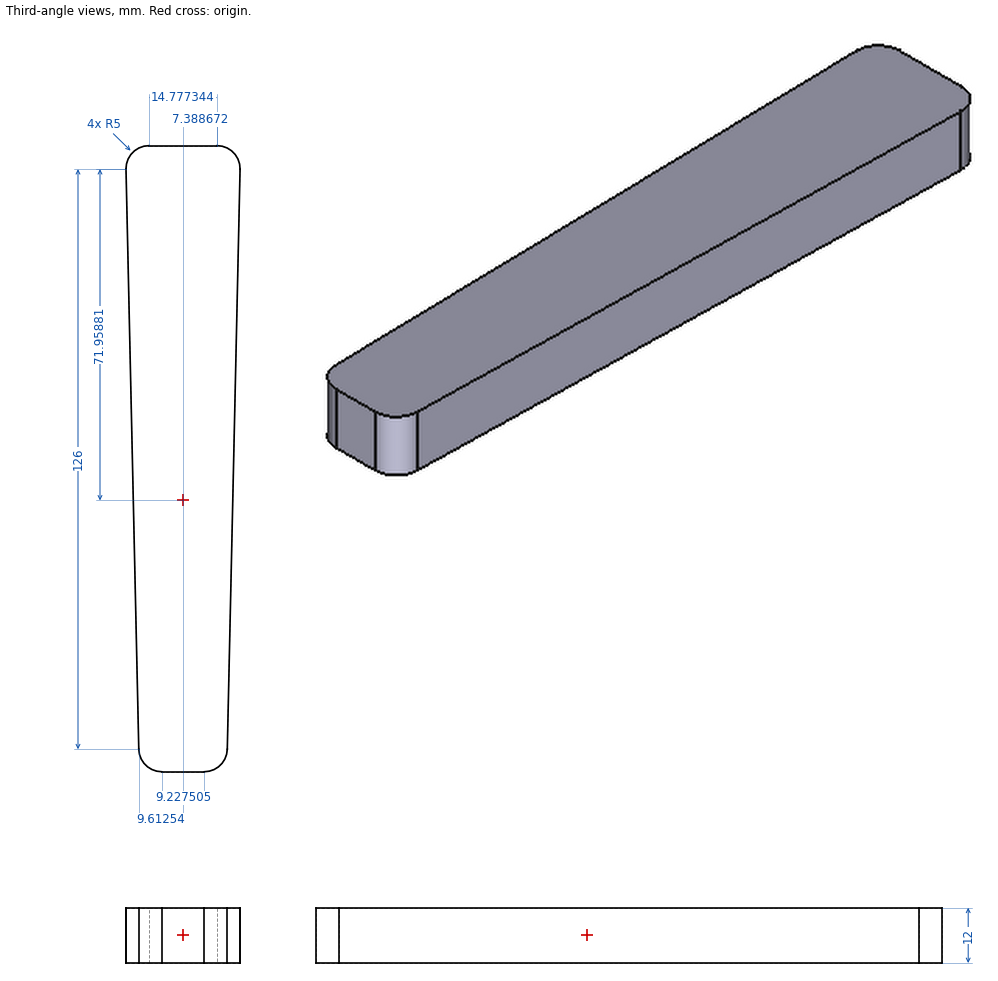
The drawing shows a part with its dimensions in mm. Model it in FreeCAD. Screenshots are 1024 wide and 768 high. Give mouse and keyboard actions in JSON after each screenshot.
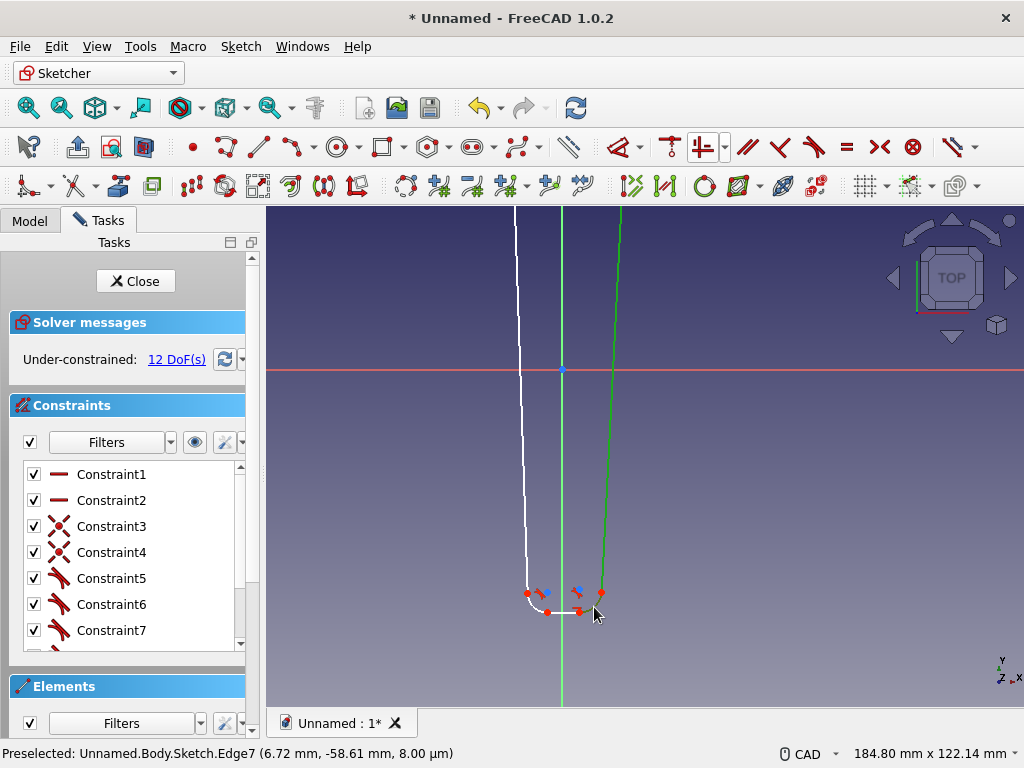
{"action": "key", "text": "t"}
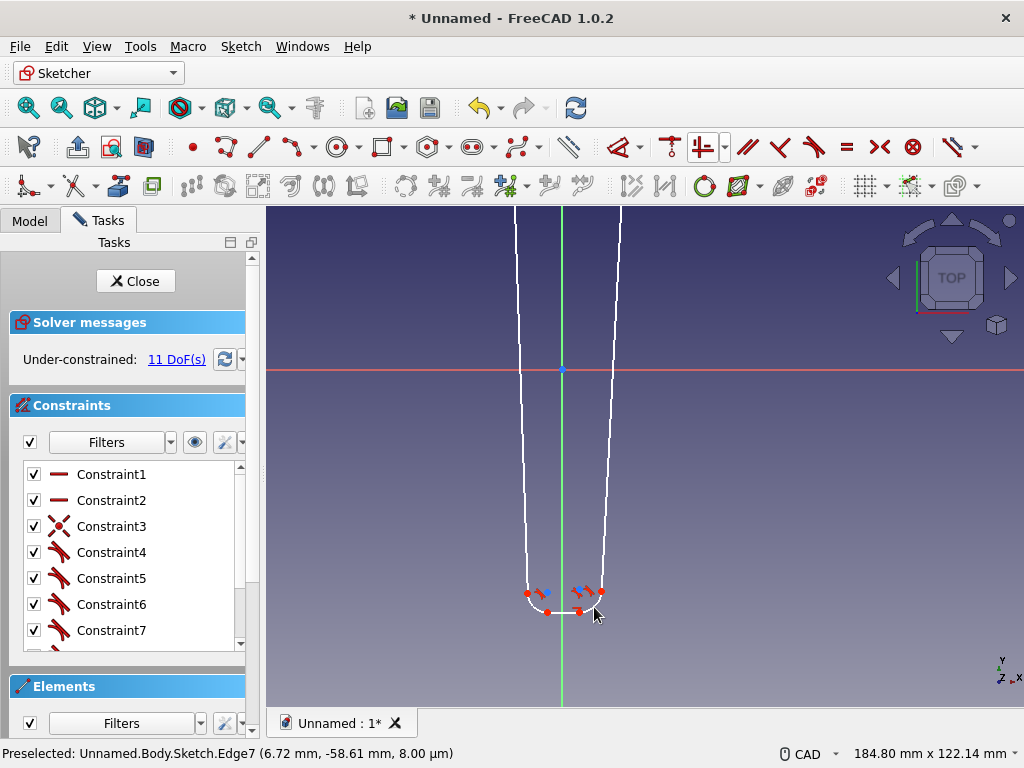
{"action": "left_click", "coordinate": [610, 436]}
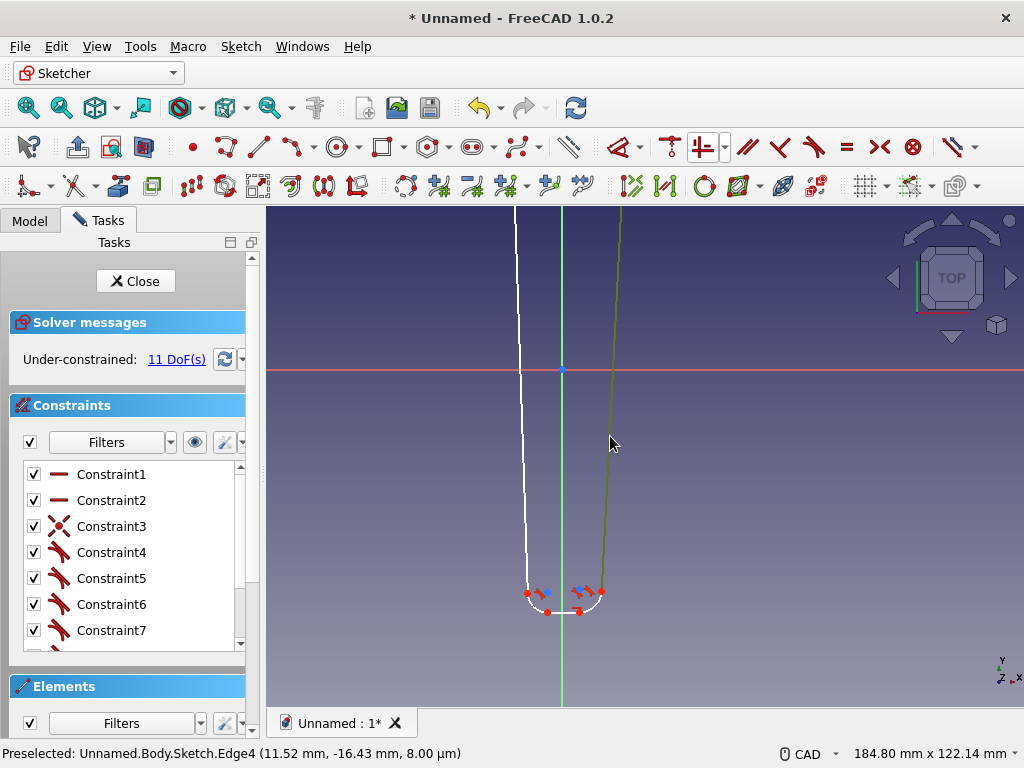
{"action": "scroll", "coordinate": [594, 607], "scroll_direction": "down", "scroll_amount": 3}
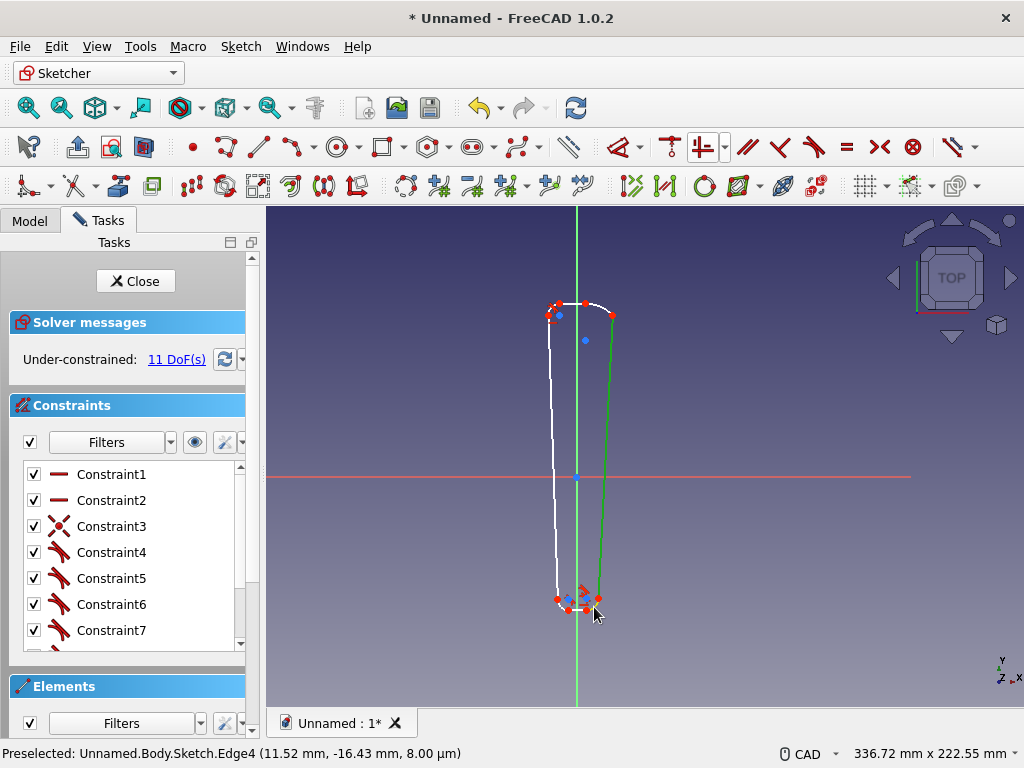
{"action": "scroll", "coordinate": [606, 310], "scroll_direction": "up", "scroll_amount": 3}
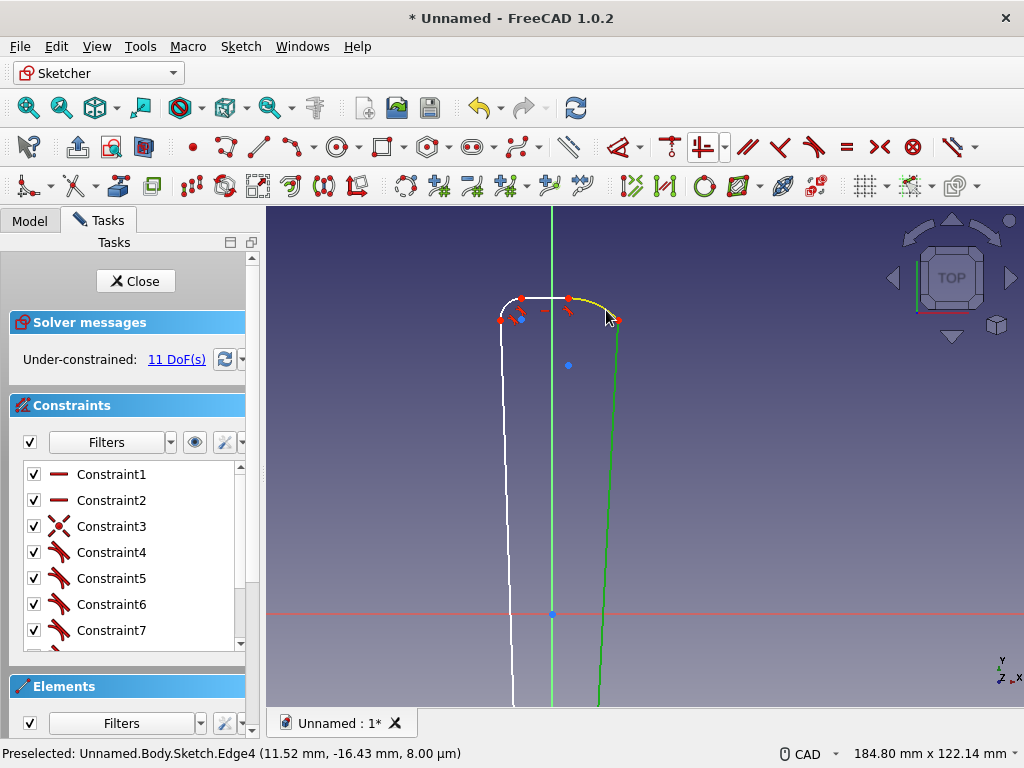
{"action": "left_click", "coordinate": [606, 309]}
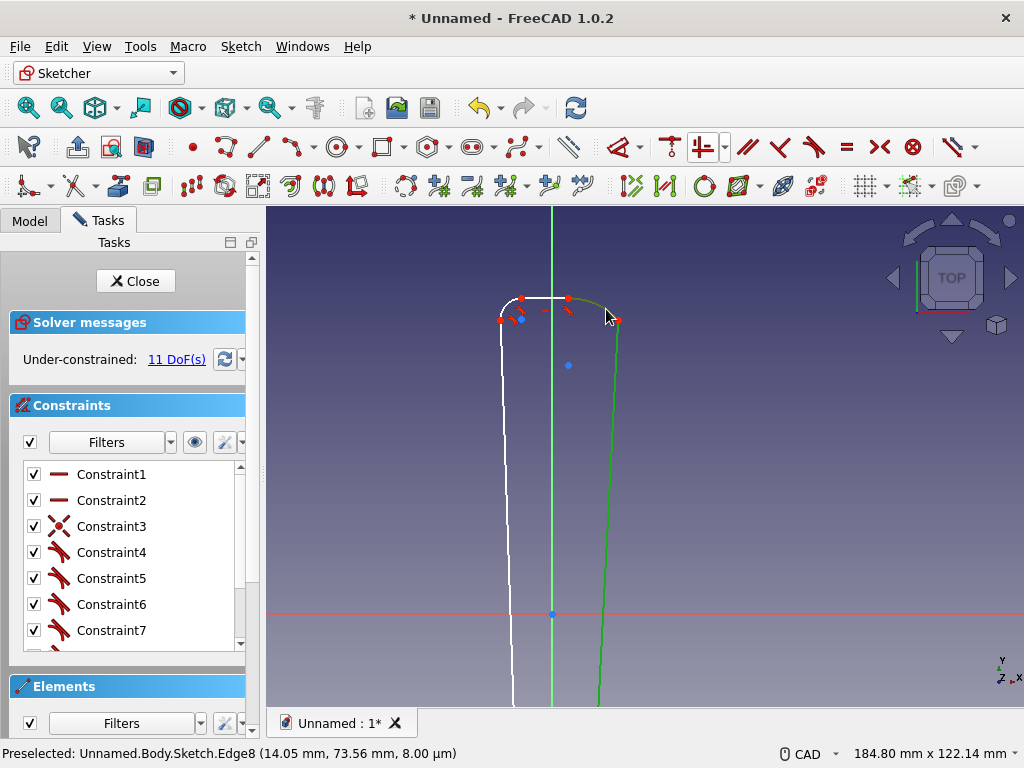
{"action": "key", "text": "t"}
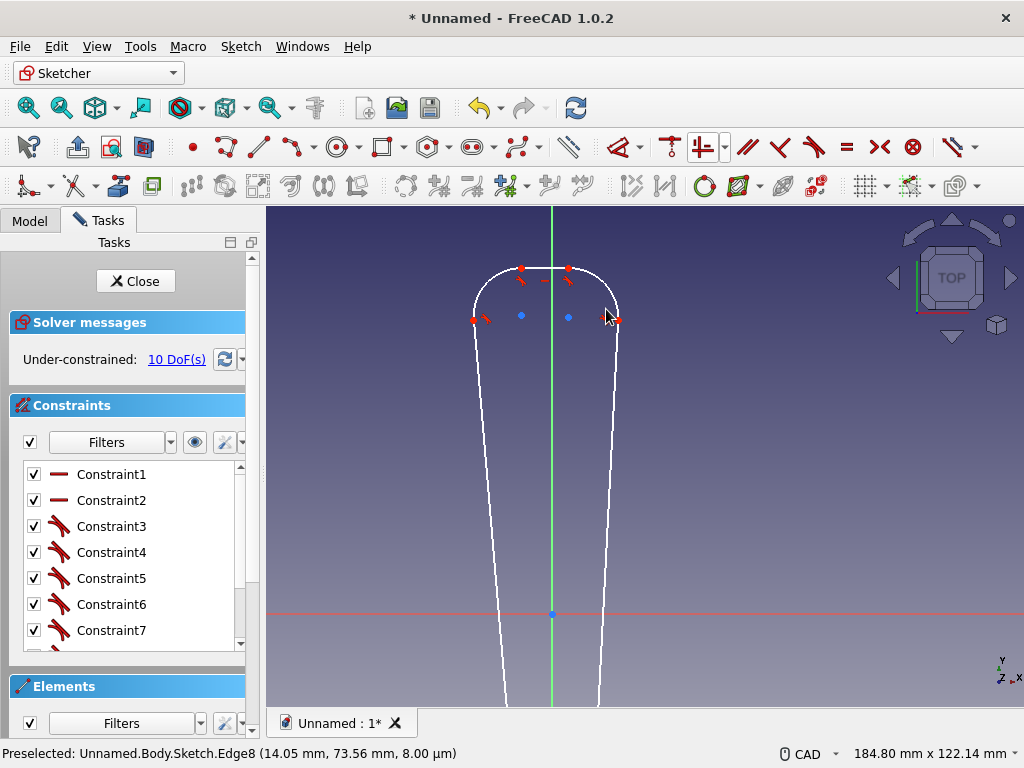
{"action": "left_click", "coordinate": [499, 274]}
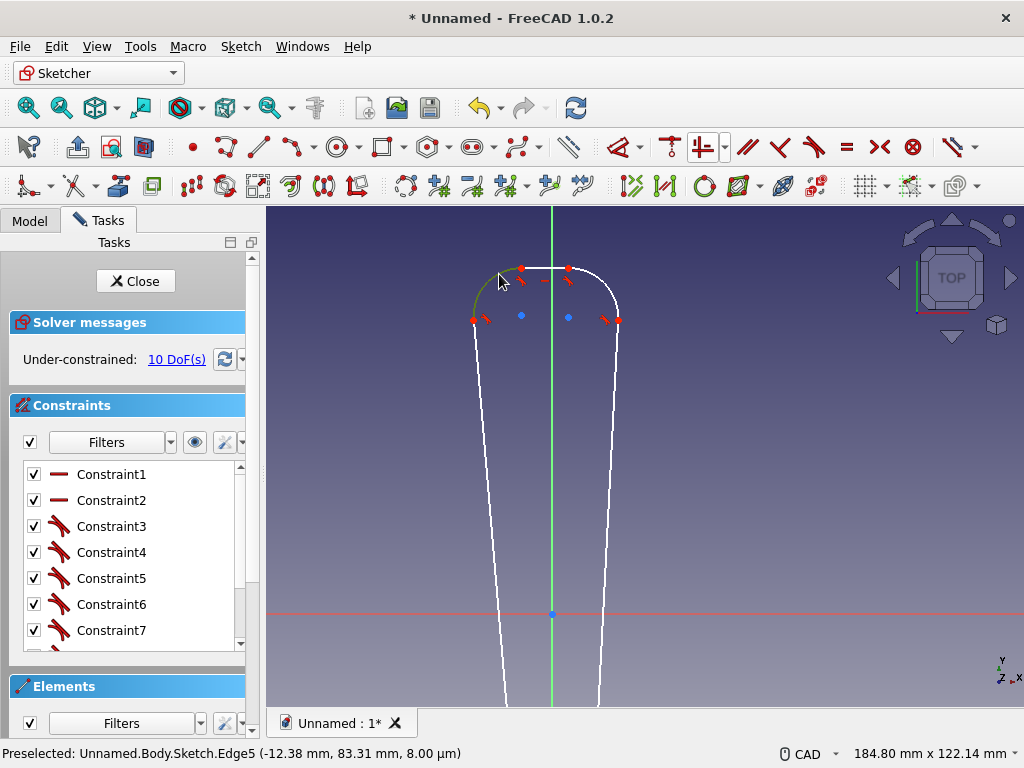
{"action": "scroll", "coordinate": [606, 310], "scroll_direction": "down", "scroll_amount": 3}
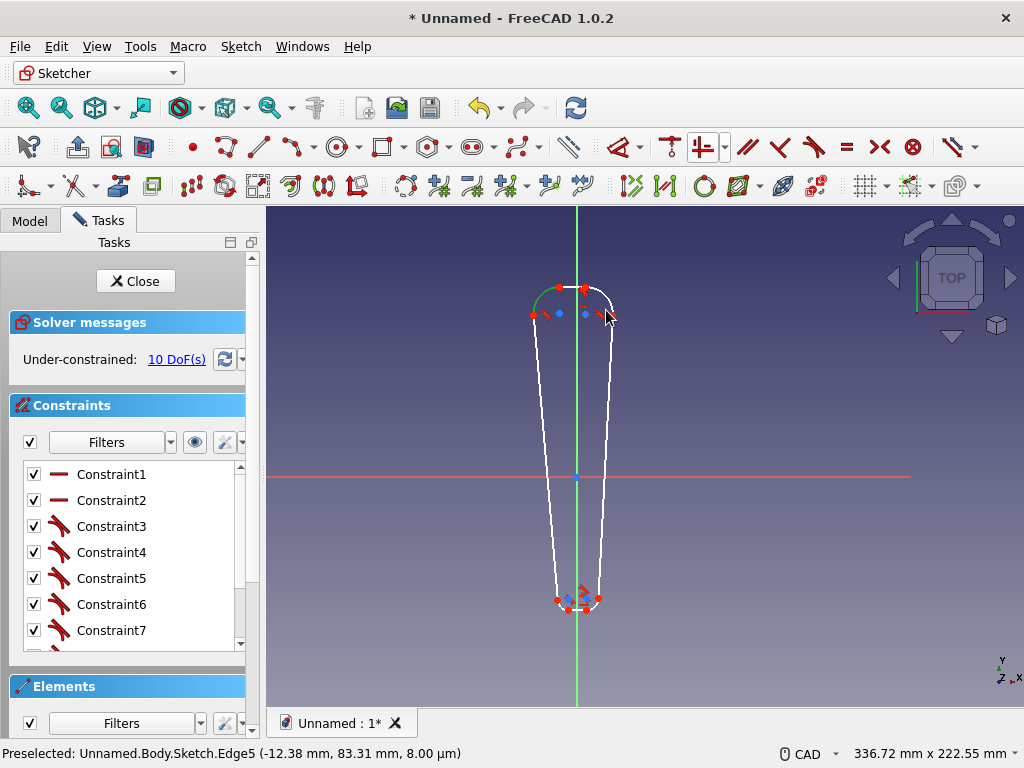
{"action": "scroll", "coordinate": [561, 608], "scroll_direction": "up", "scroll_amount": 3}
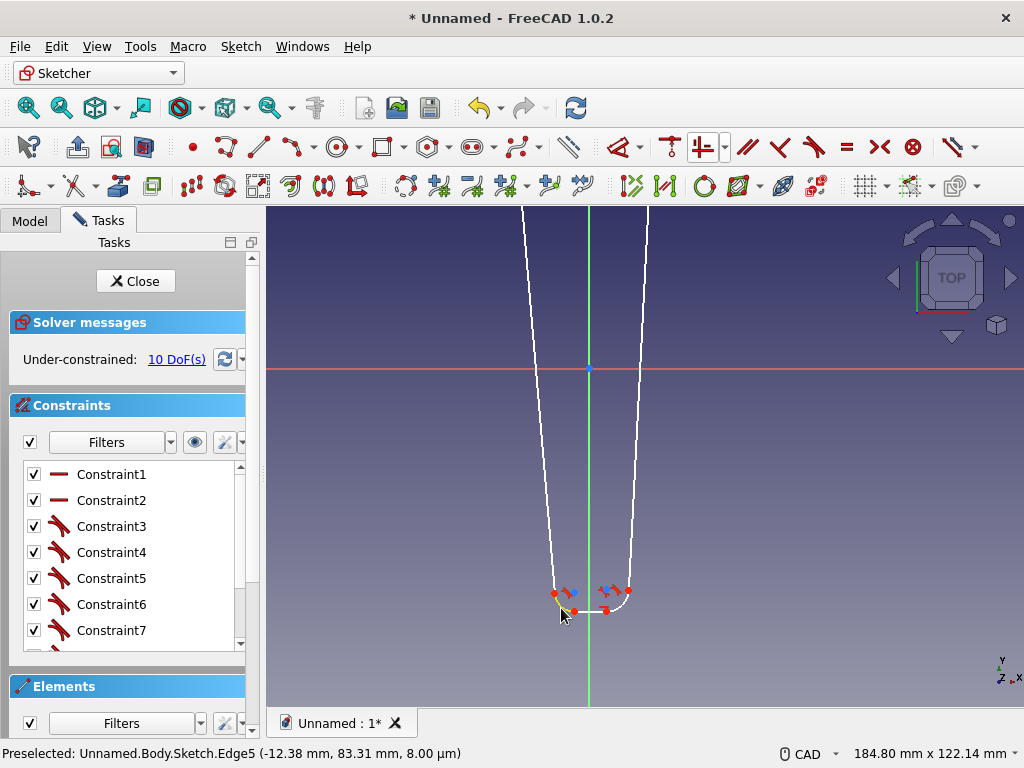
{"action": "left_click", "coordinate": [561, 607]}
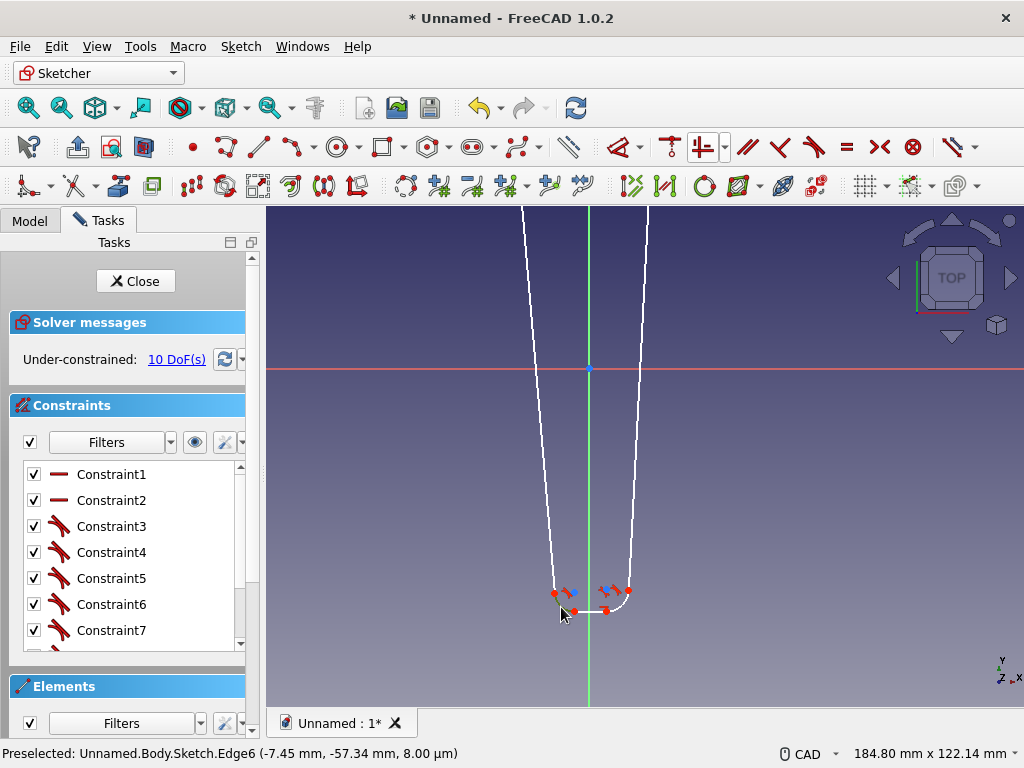
{"action": "scroll", "coordinate": [616, 609], "scroll_direction": "up", "scroll_amount": 2}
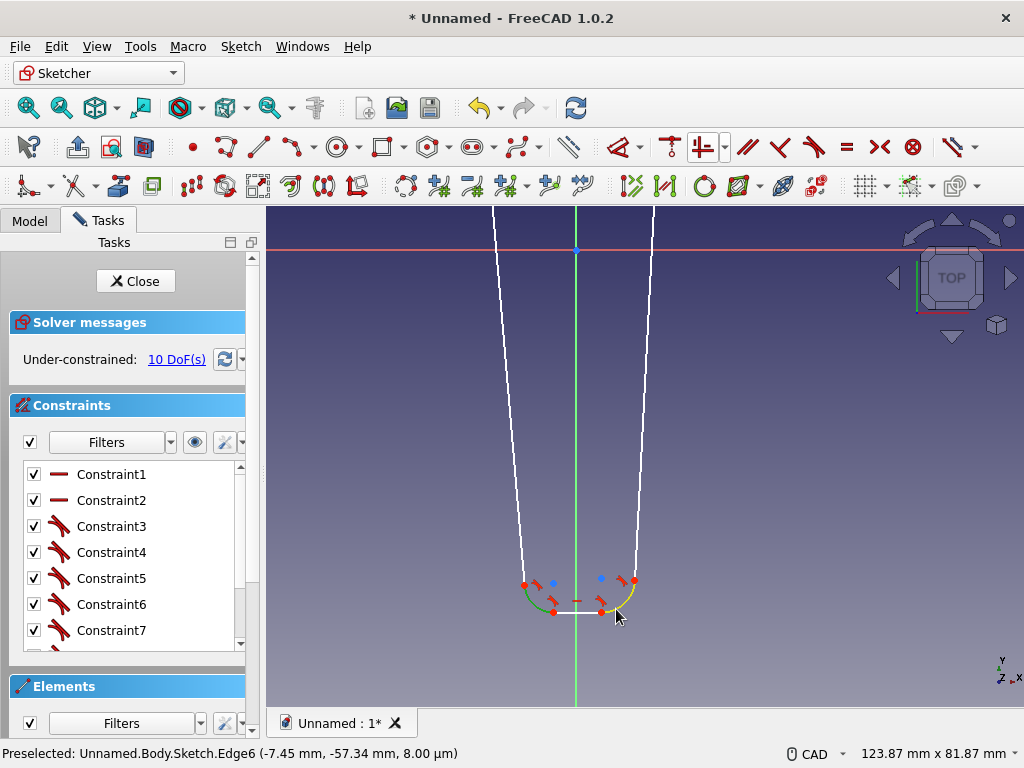
{"action": "left_click", "coordinate": [616, 609]}